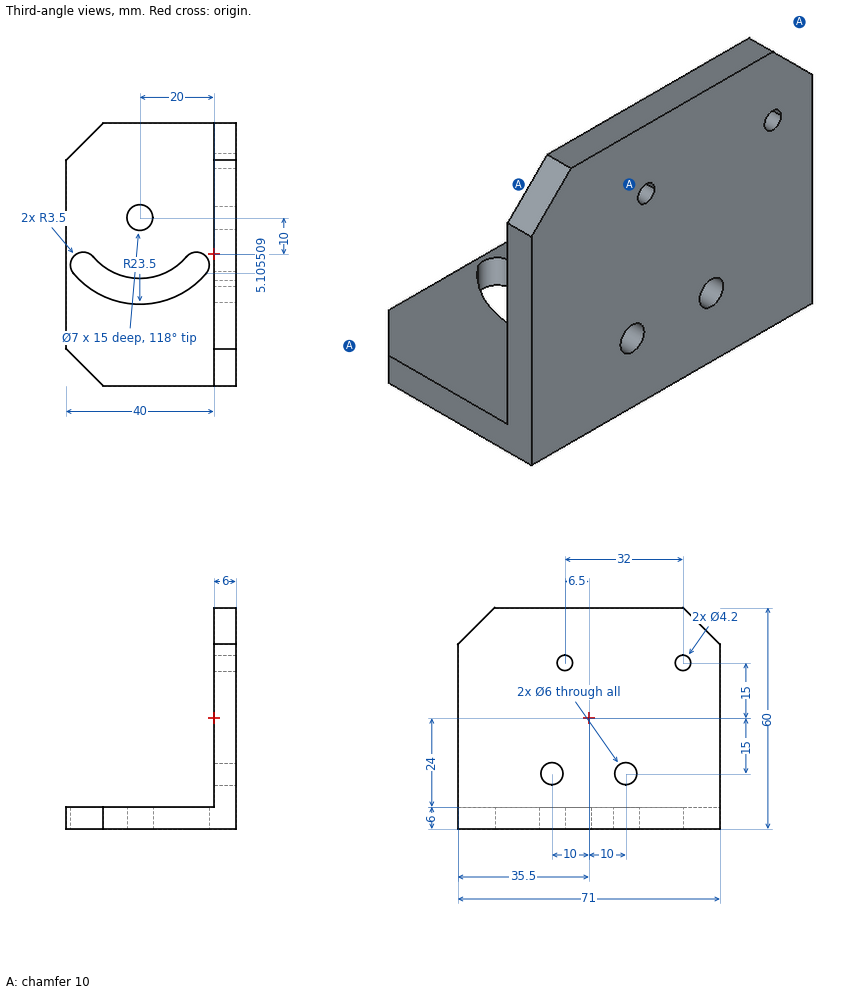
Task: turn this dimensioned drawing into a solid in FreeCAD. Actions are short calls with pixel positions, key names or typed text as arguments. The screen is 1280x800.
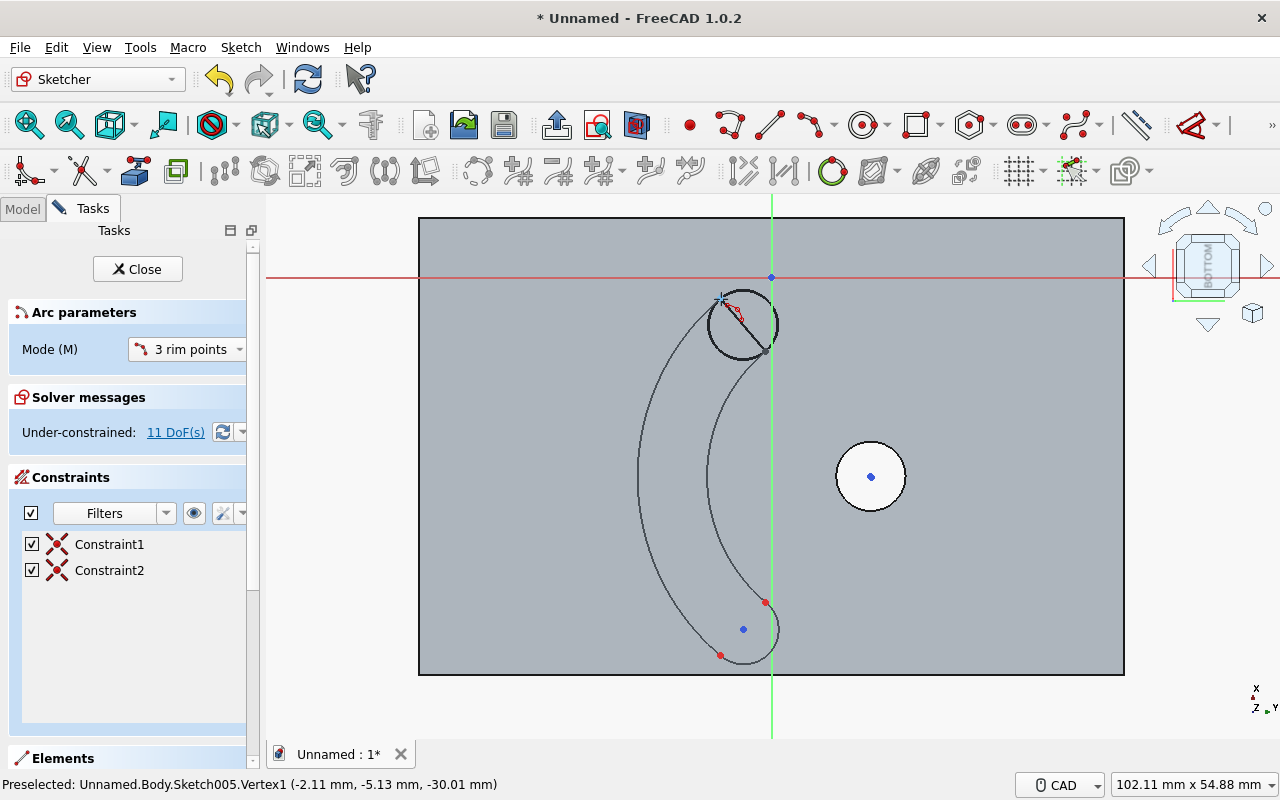
scroll(752, 290, up, 2)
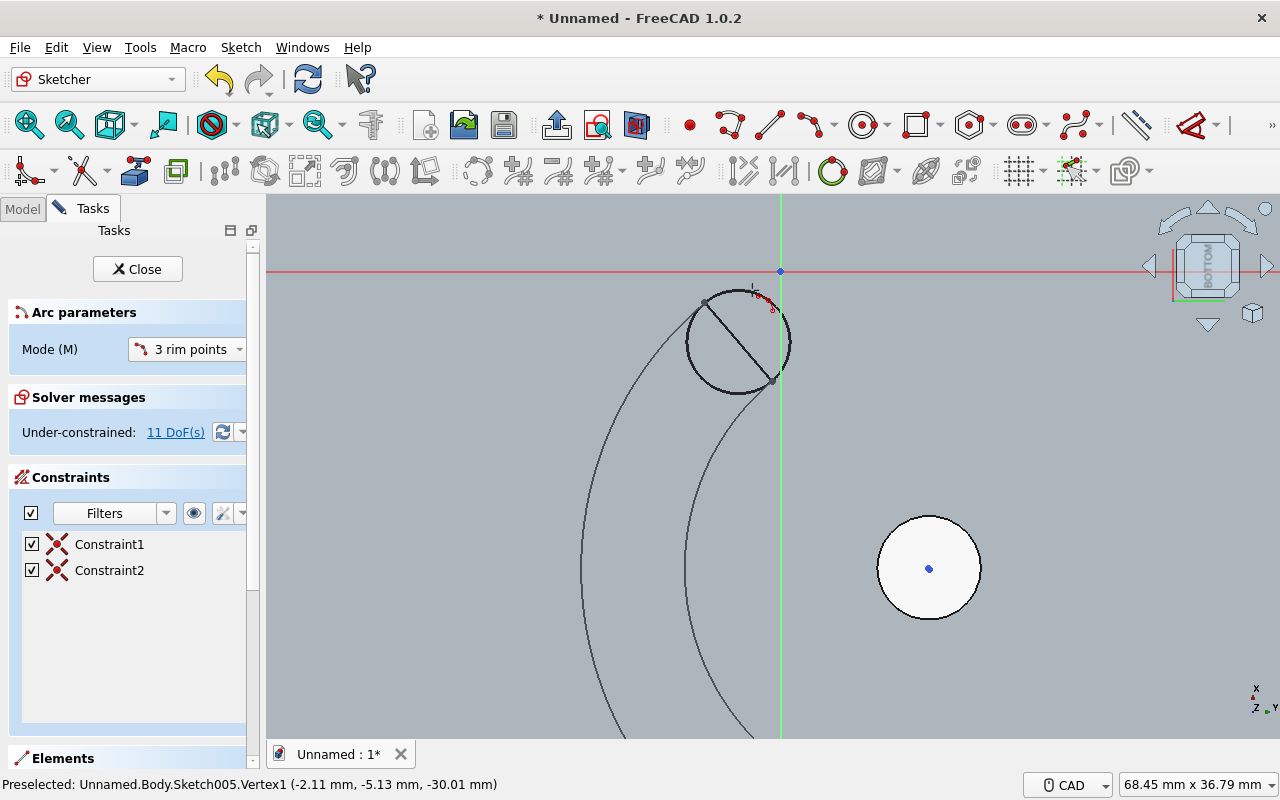
click(751, 291)
key(Escape)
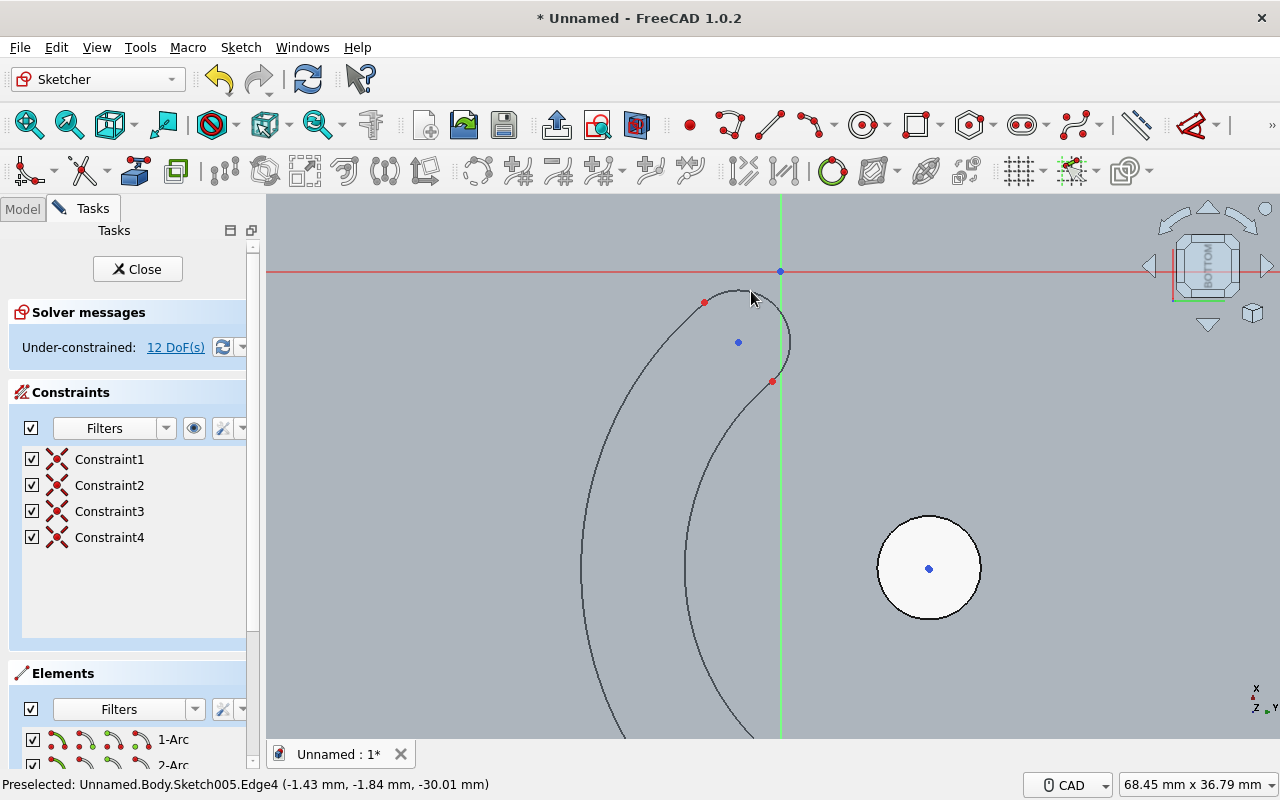
click(602, 450)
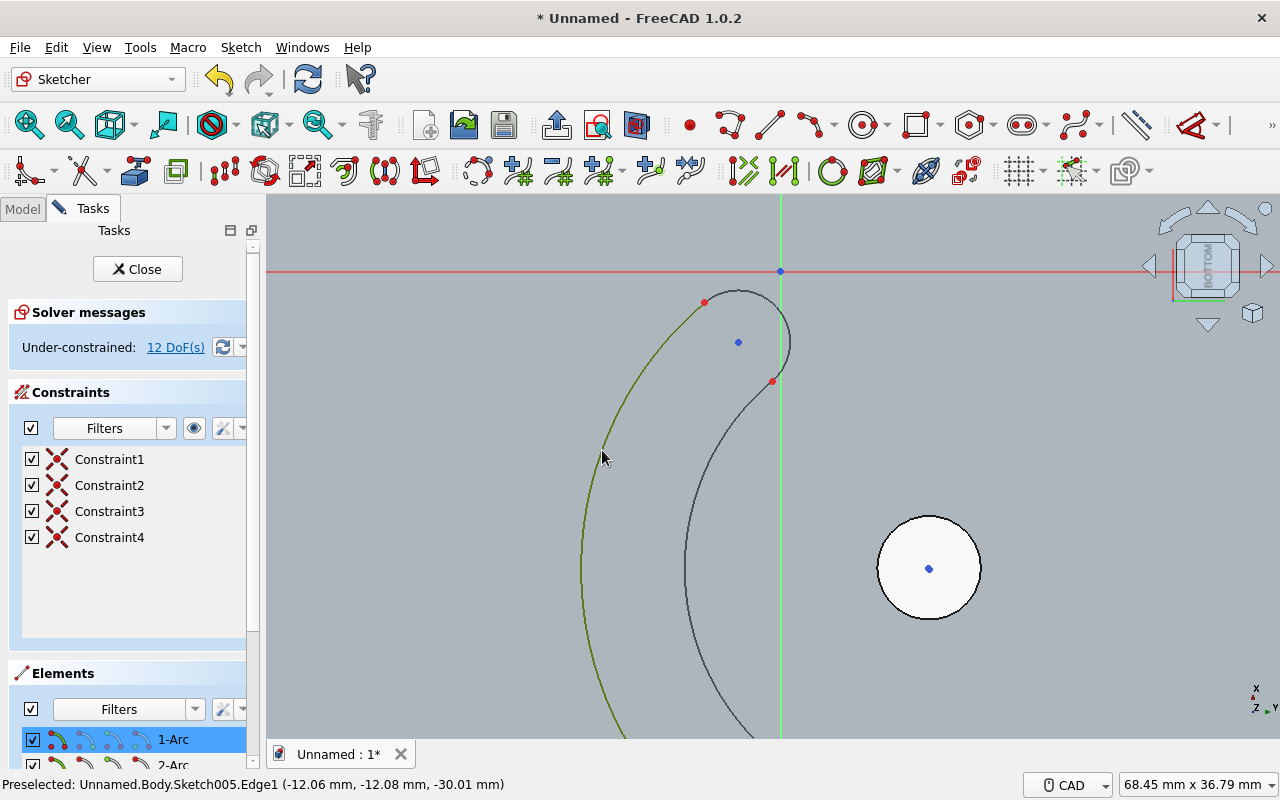
scroll(752, 291, down, 2)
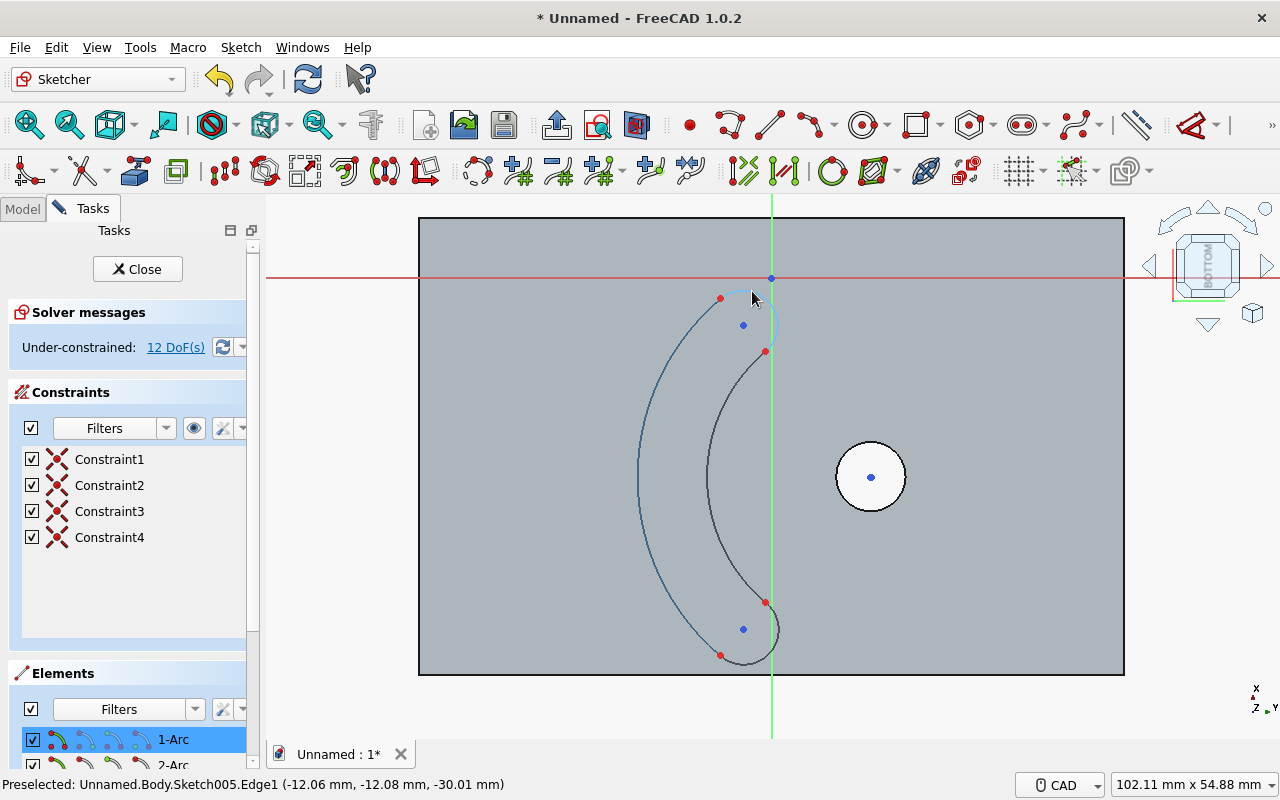
click(752, 664)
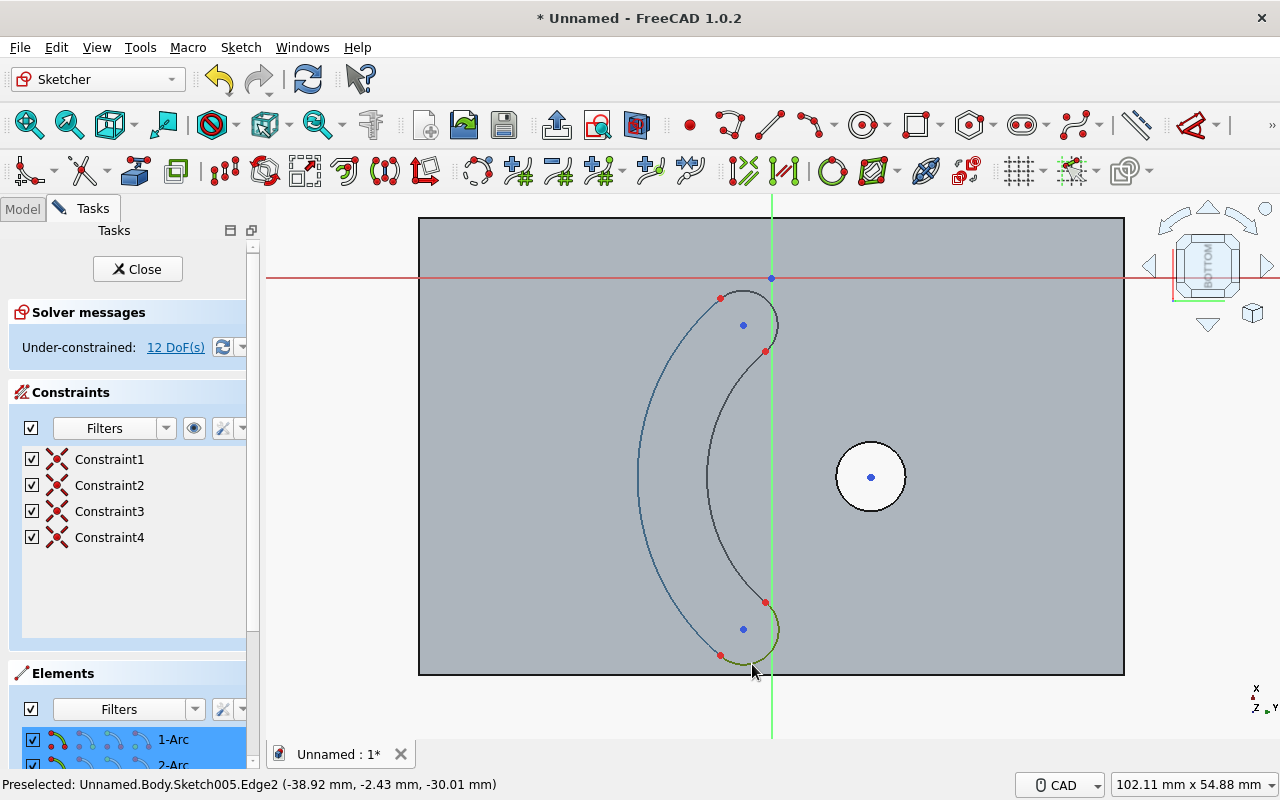
key(t)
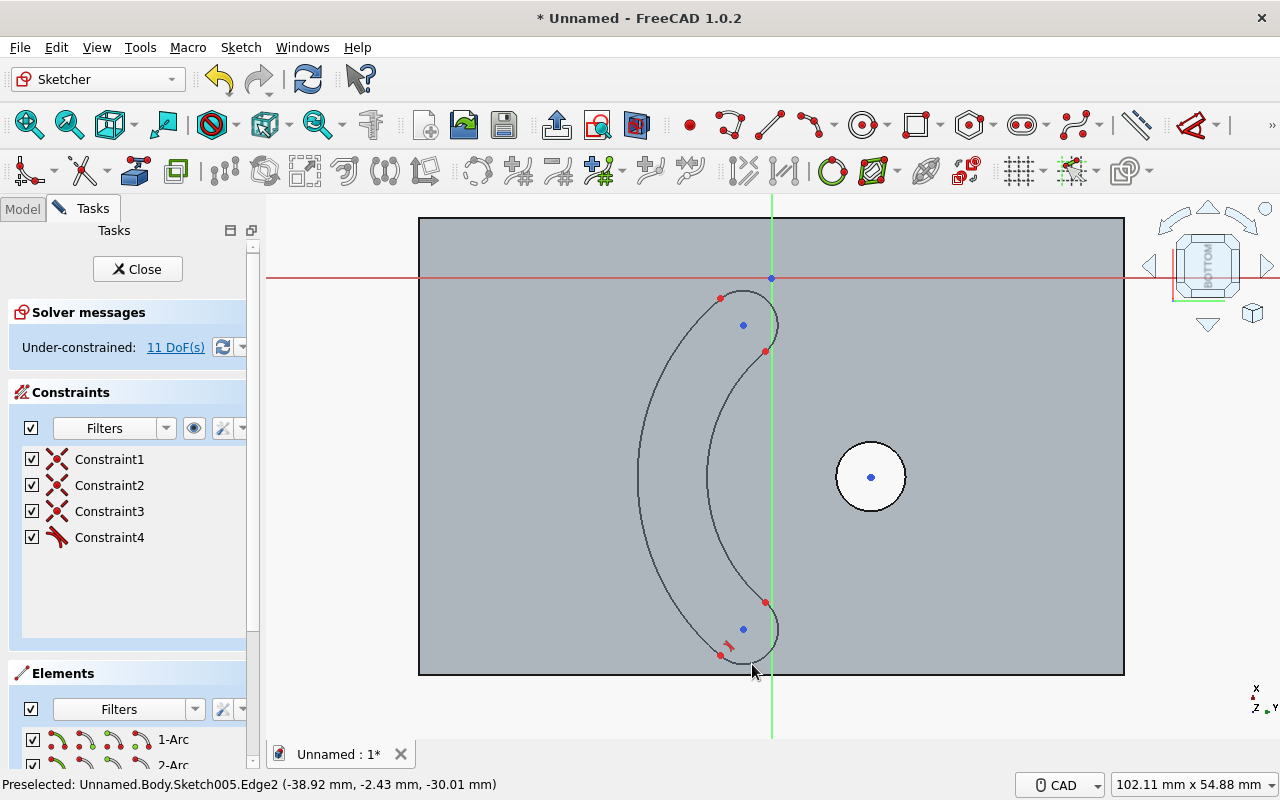
click(652, 398)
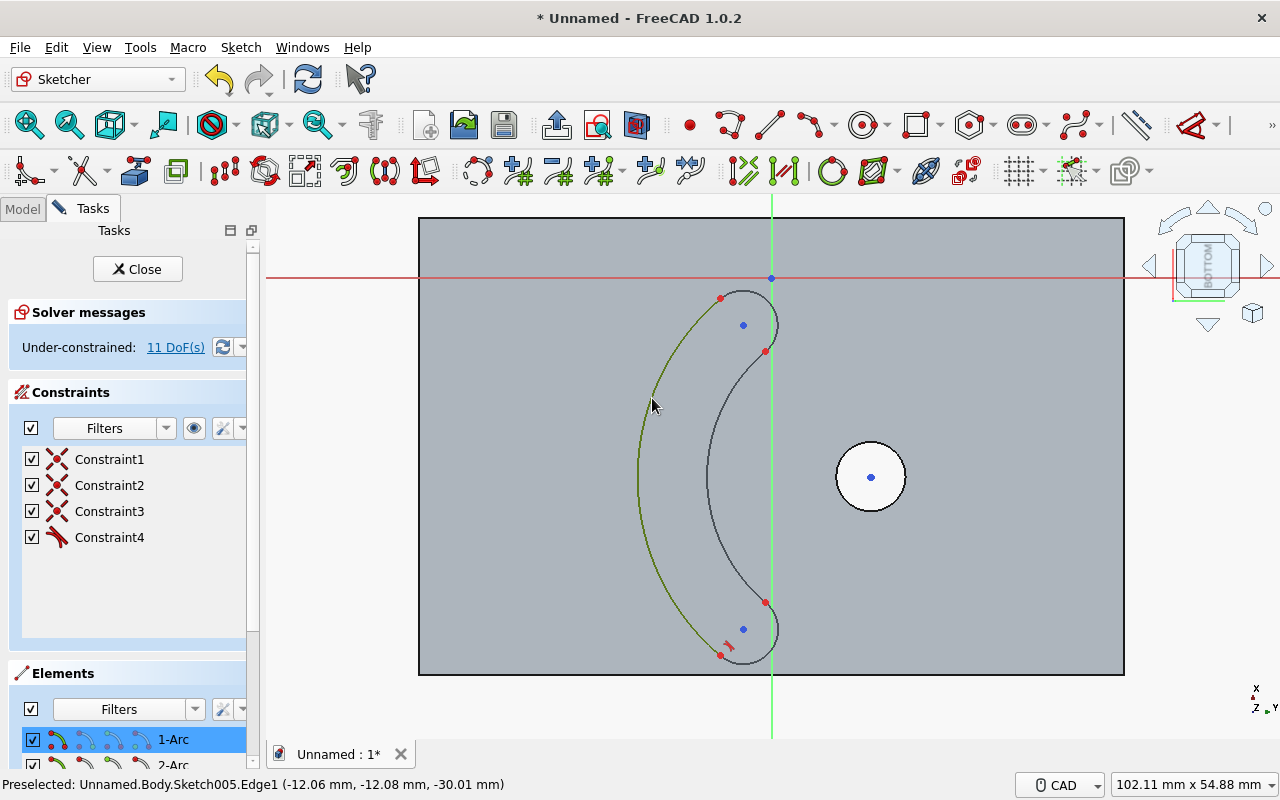
click(751, 292)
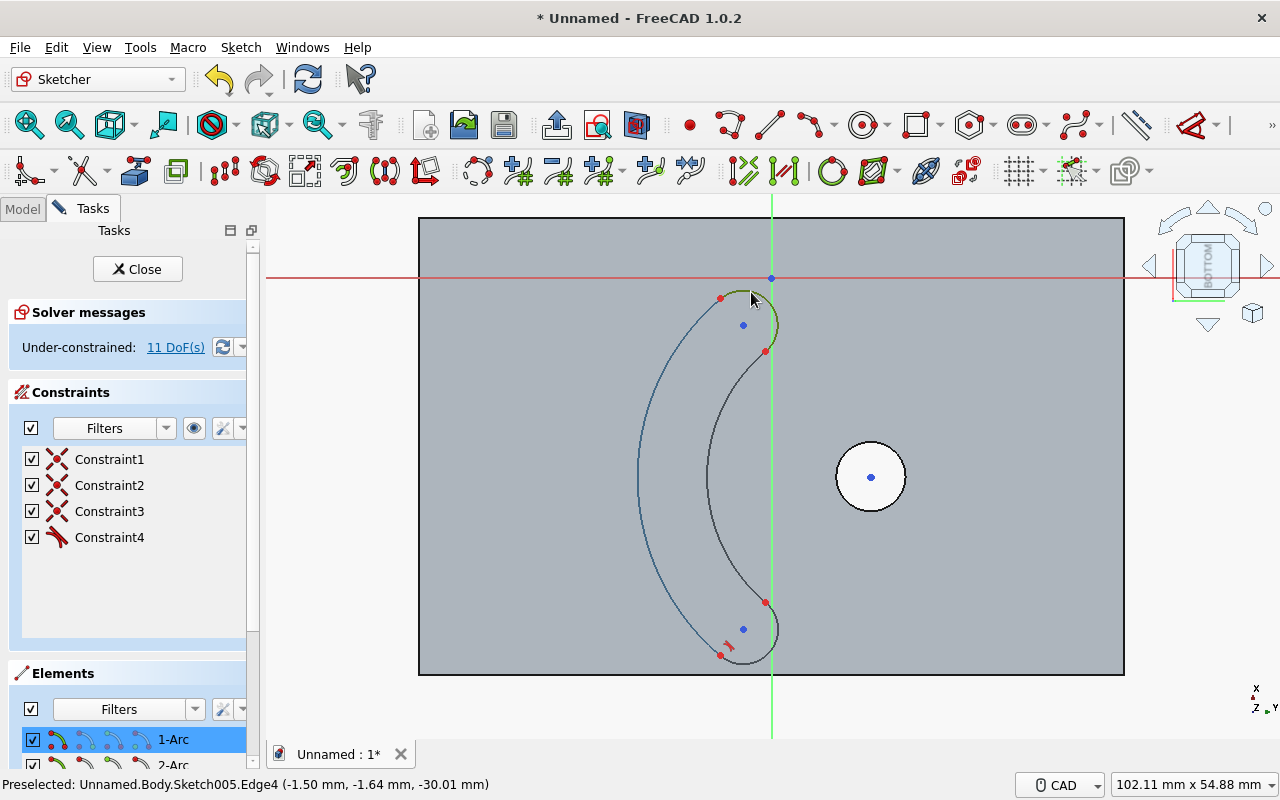
key(t)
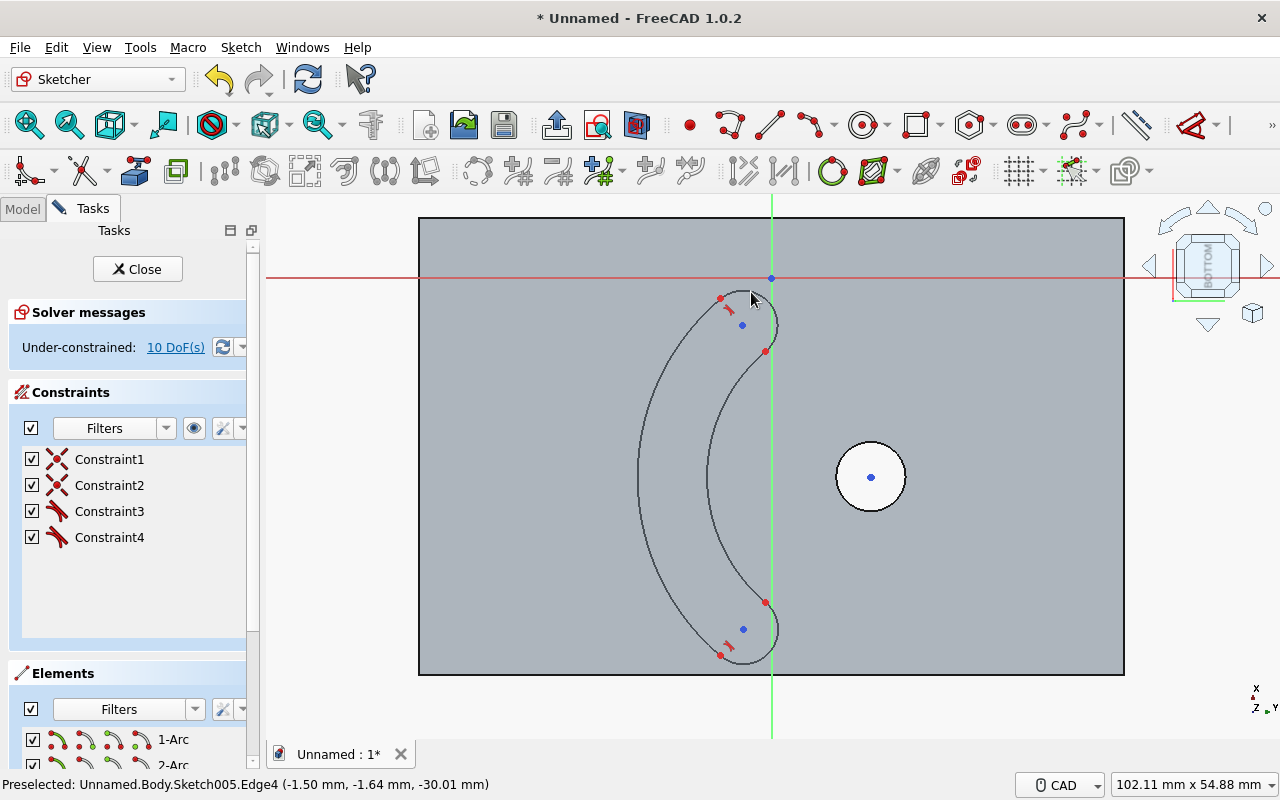
click(752, 663)